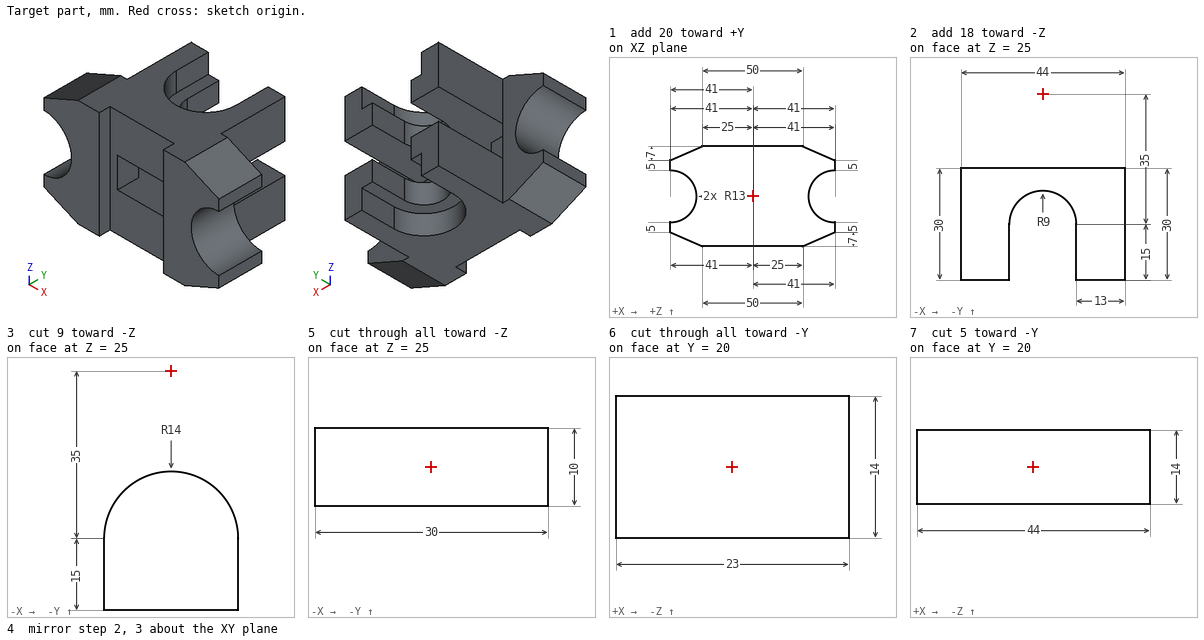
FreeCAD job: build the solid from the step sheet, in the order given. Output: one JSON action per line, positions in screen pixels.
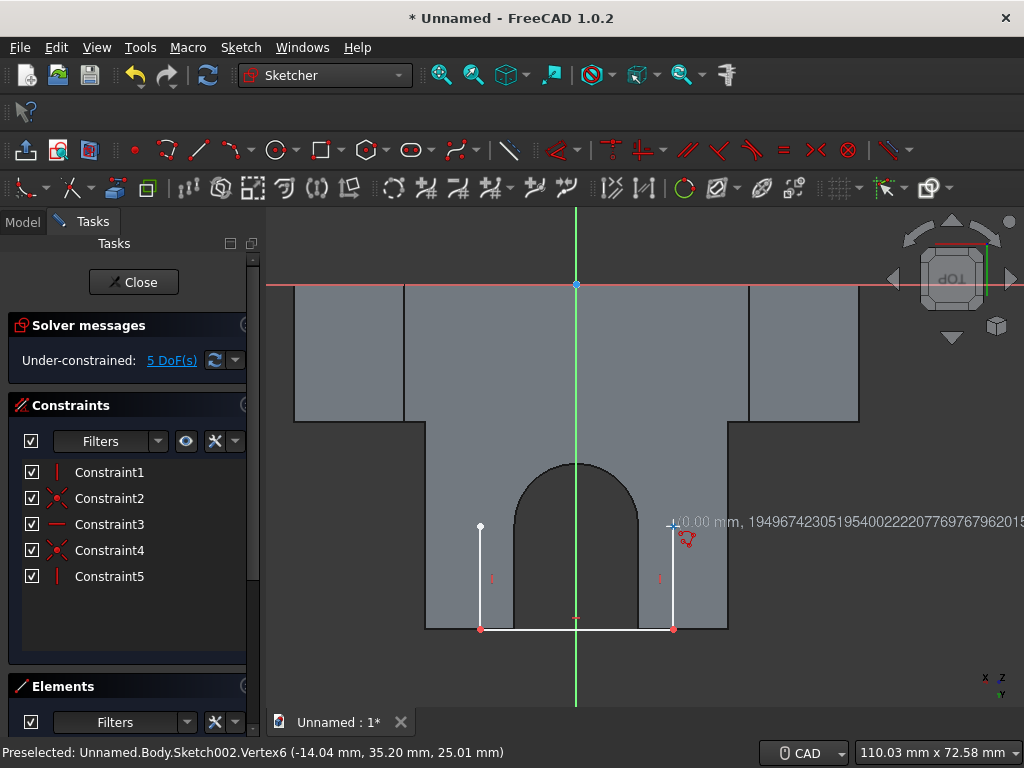
{"action": "left_click", "coordinate": [232, 150]}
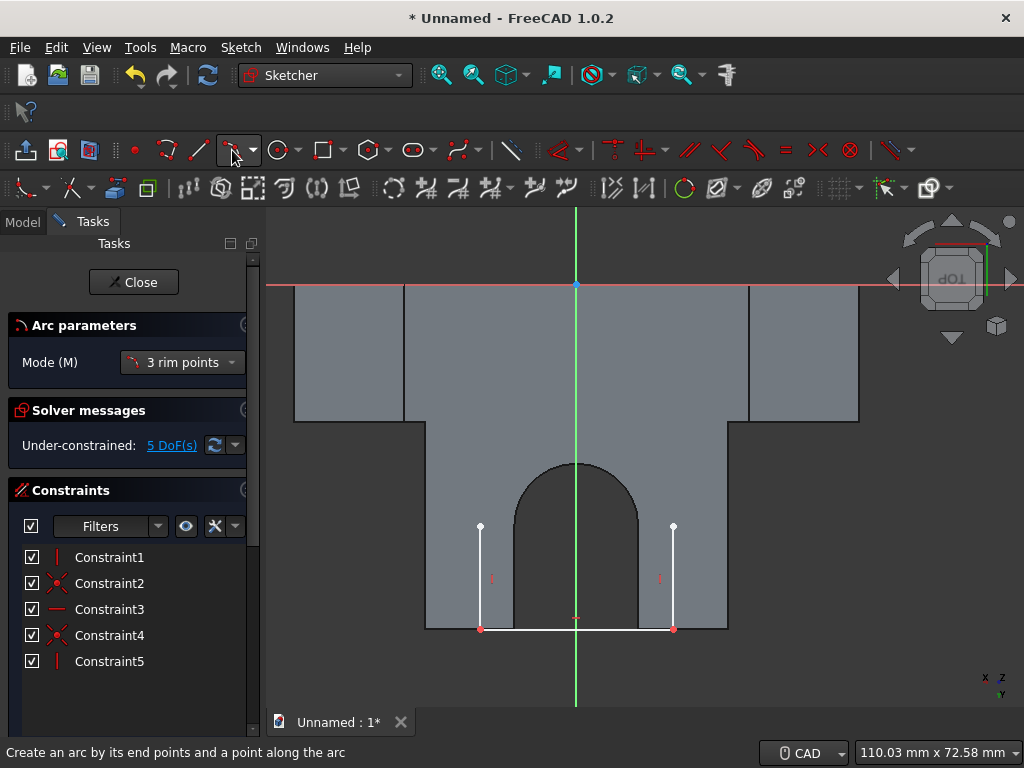
{"action": "left_click", "coordinate": [673, 527]}
{"action": "left_click", "coordinate": [480, 527]}
{"action": "left_click", "coordinate": [606, 434]}
{"action": "key", "text": "Escape"}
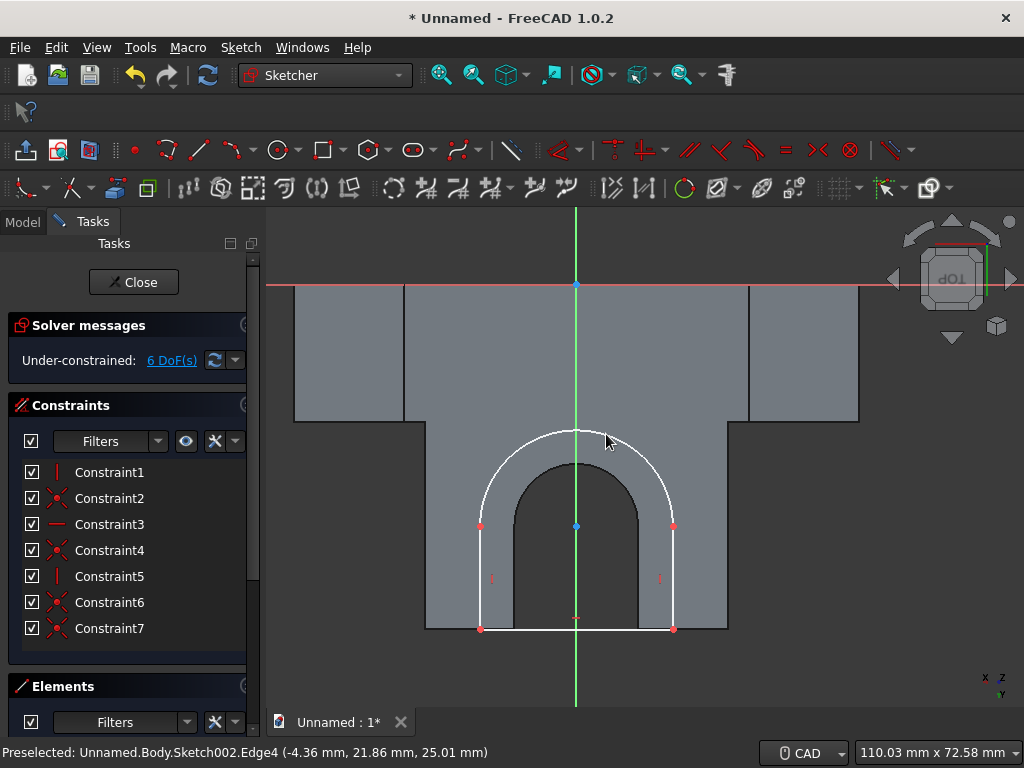
{"action": "left_click", "coordinate": [480, 558]}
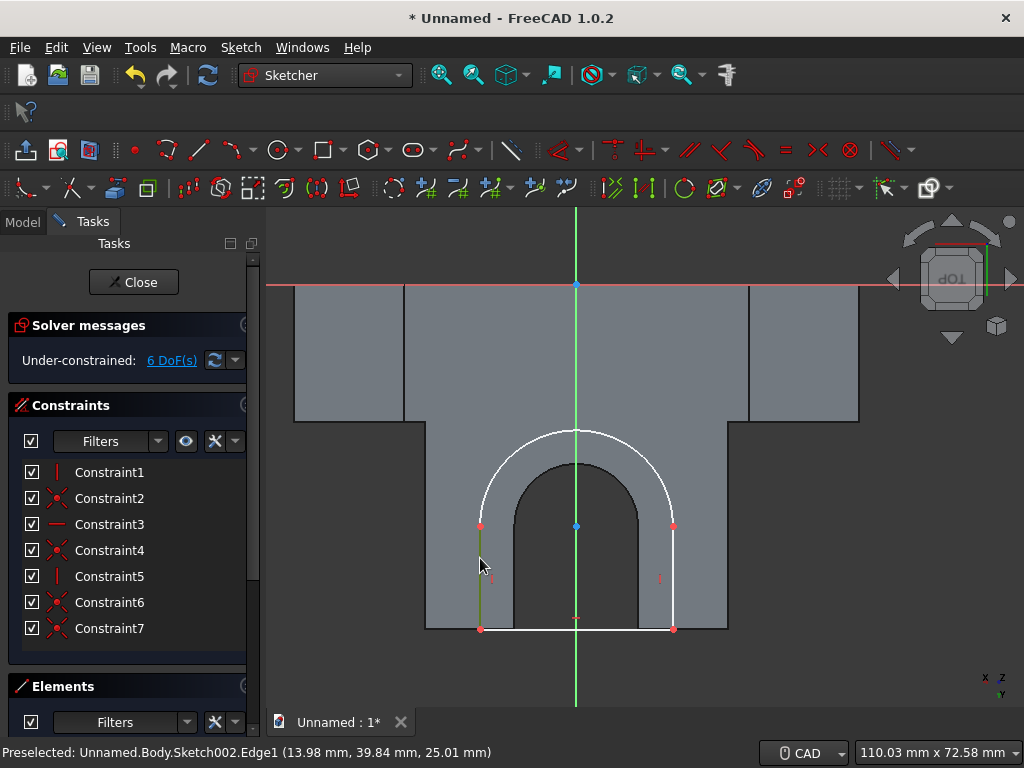
{"action": "left_click", "coordinate": [633, 449]}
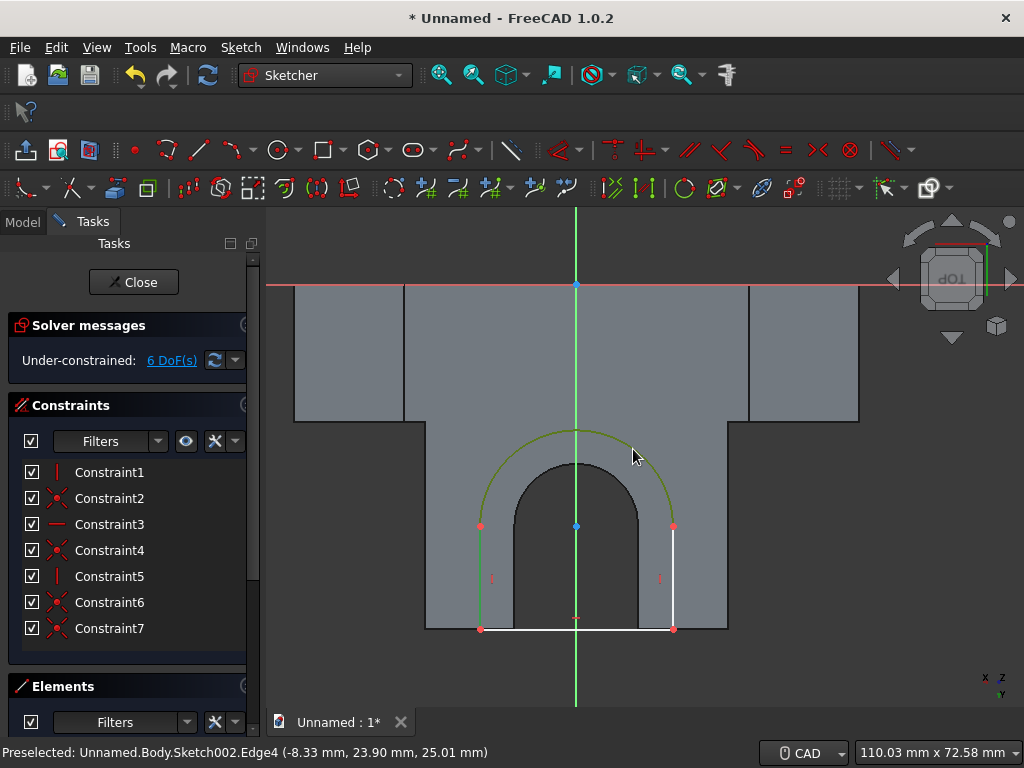
{"action": "left_click", "coordinate": [754, 150]}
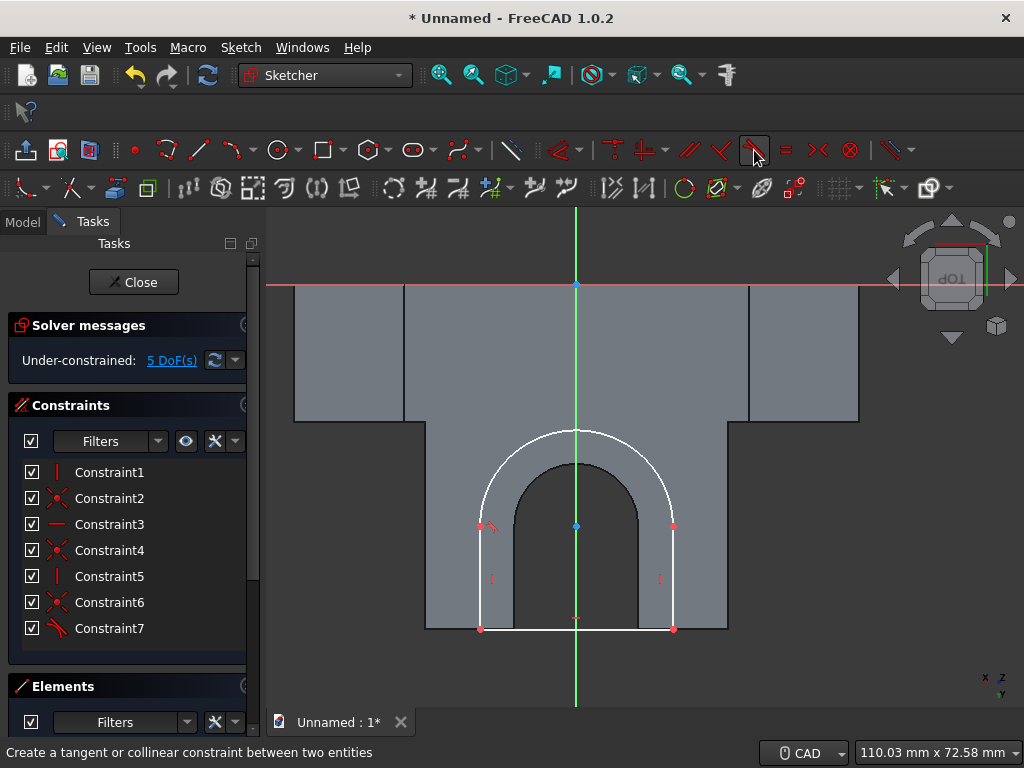
{"action": "left_click", "coordinate": [673, 599]}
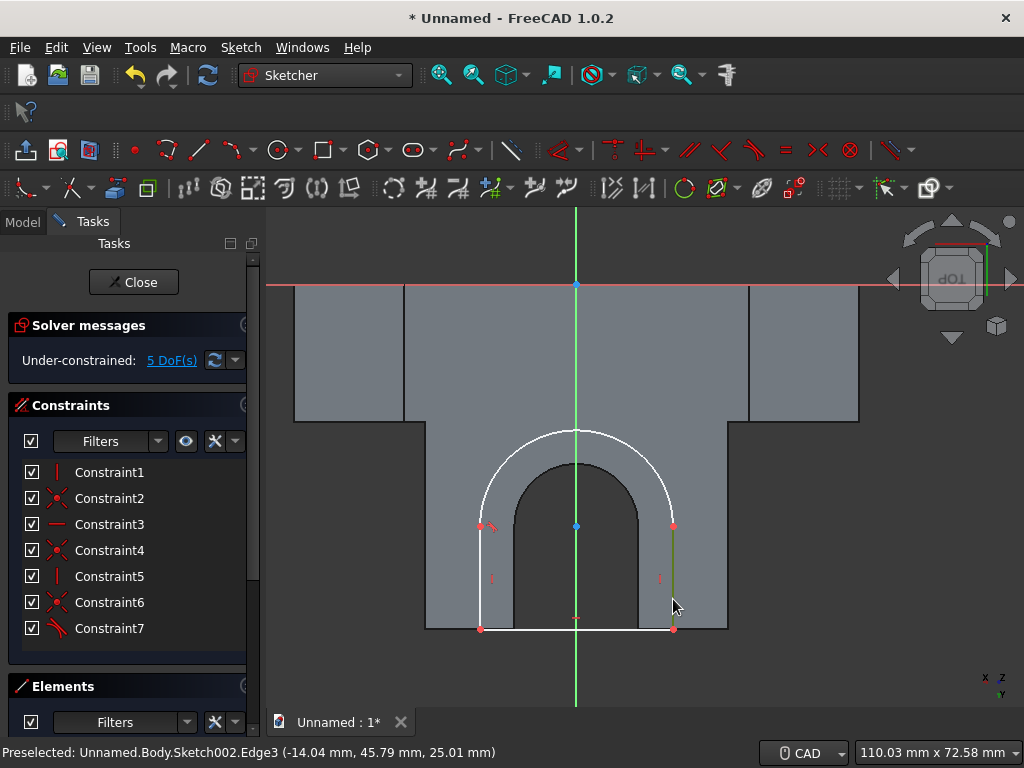
{"action": "left_click", "coordinate": [633, 449]}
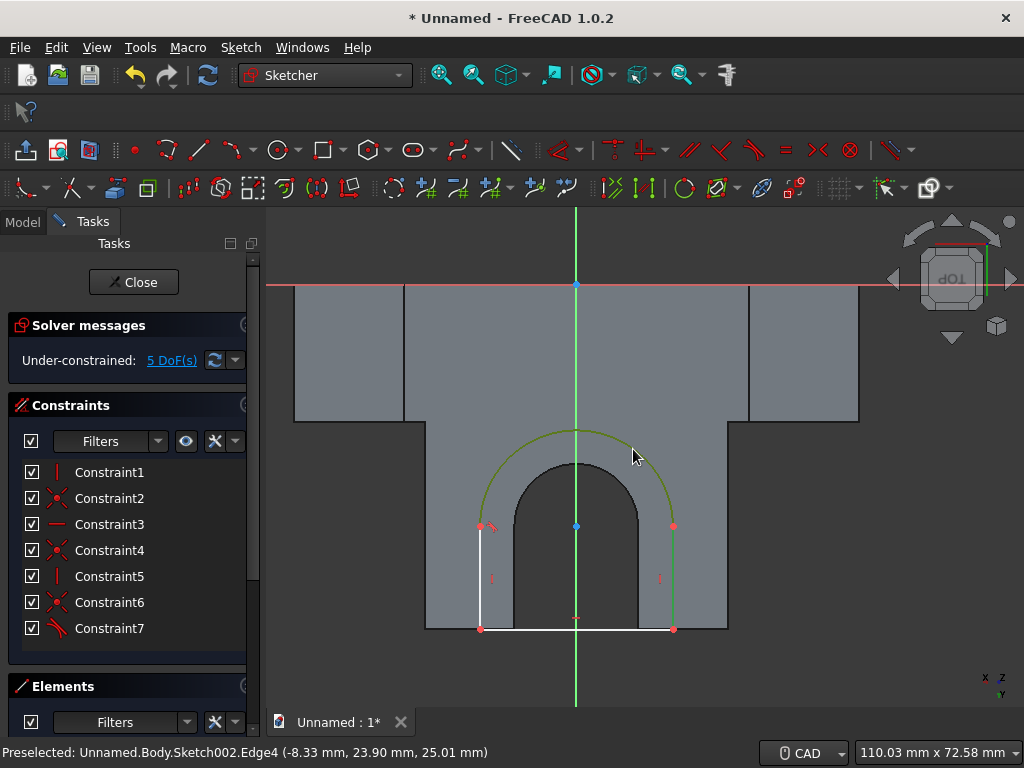
{"action": "left_click", "coordinate": [754, 150]}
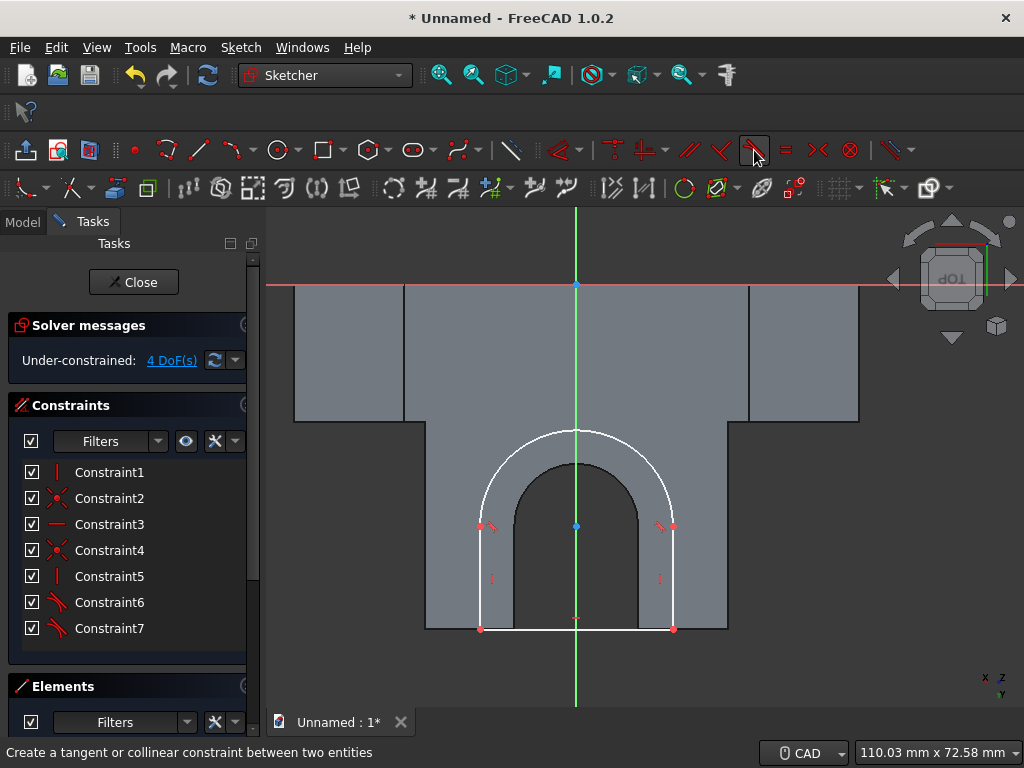
{"action": "left_click", "coordinate": [577, 527]}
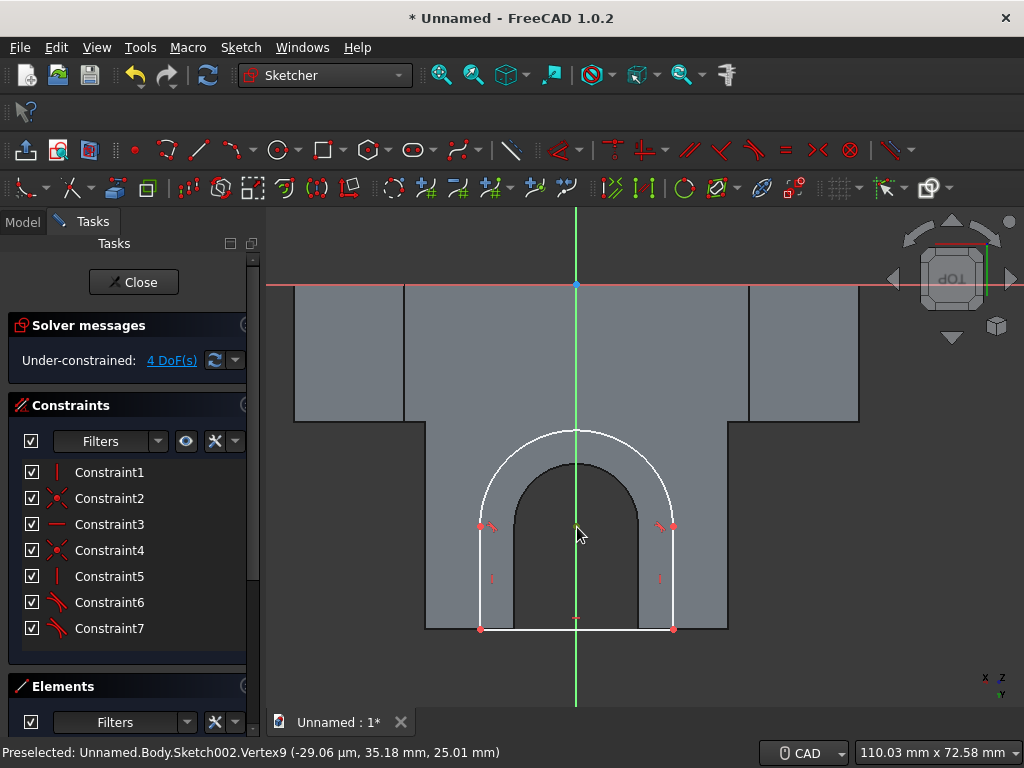
{"action": "left_click", "coordinate": [576, 584]}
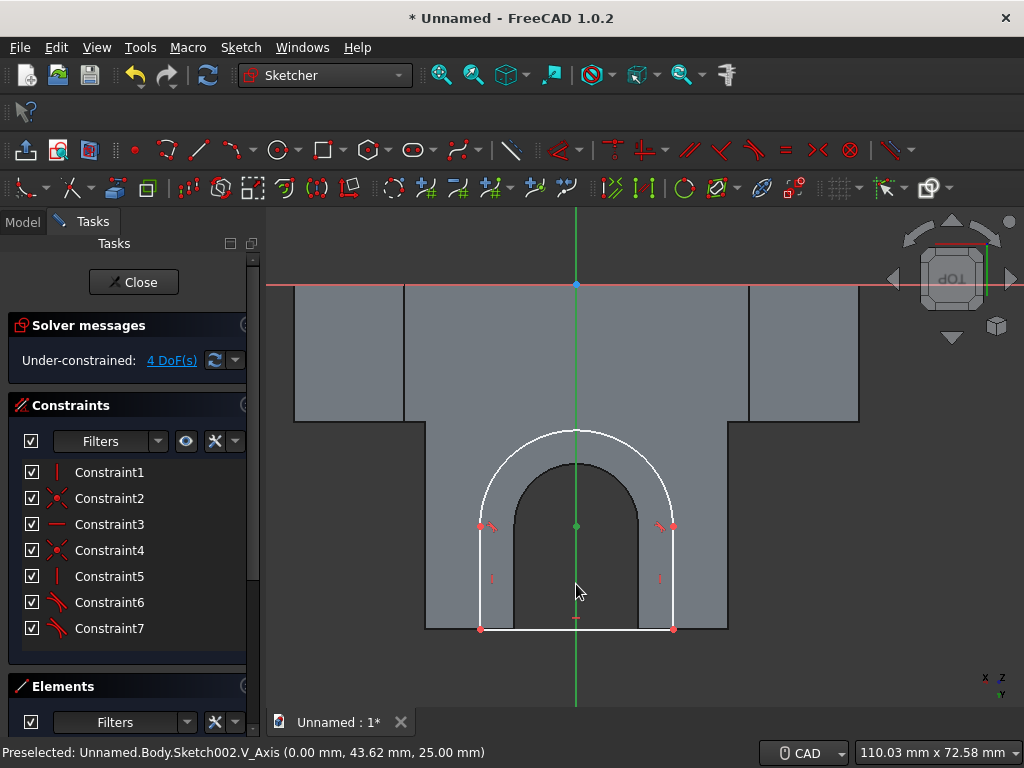
{"action": "left_click", "coordinate": [614, 150]}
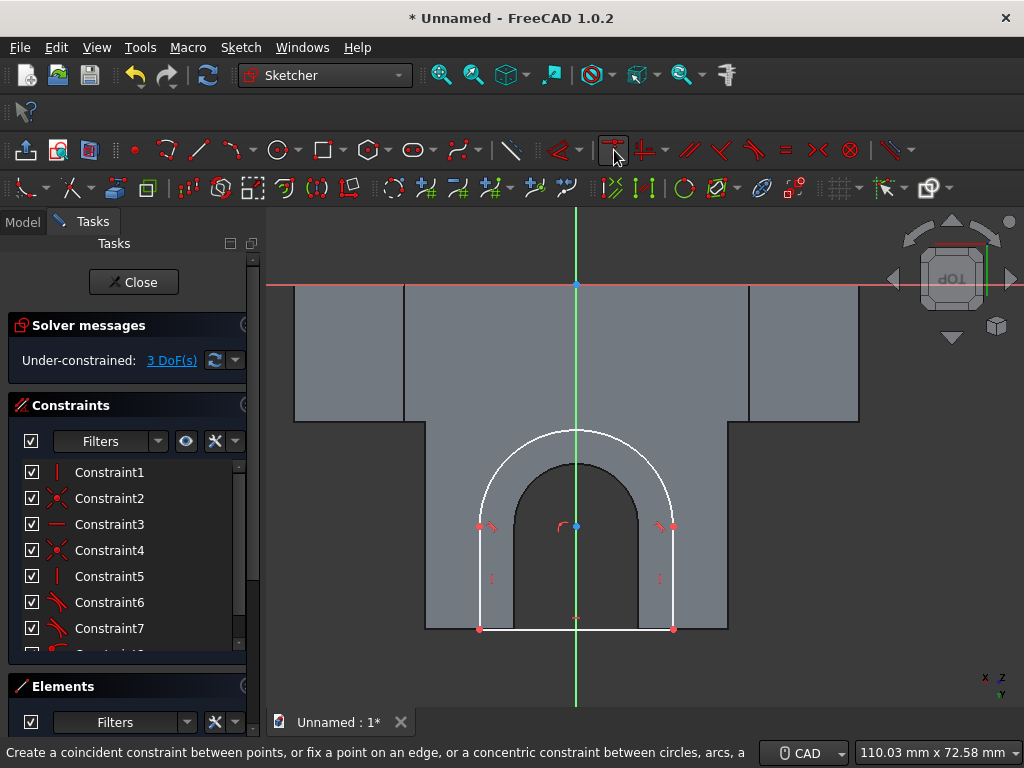
{"action": "left_click", "coordinate": [558, 150]}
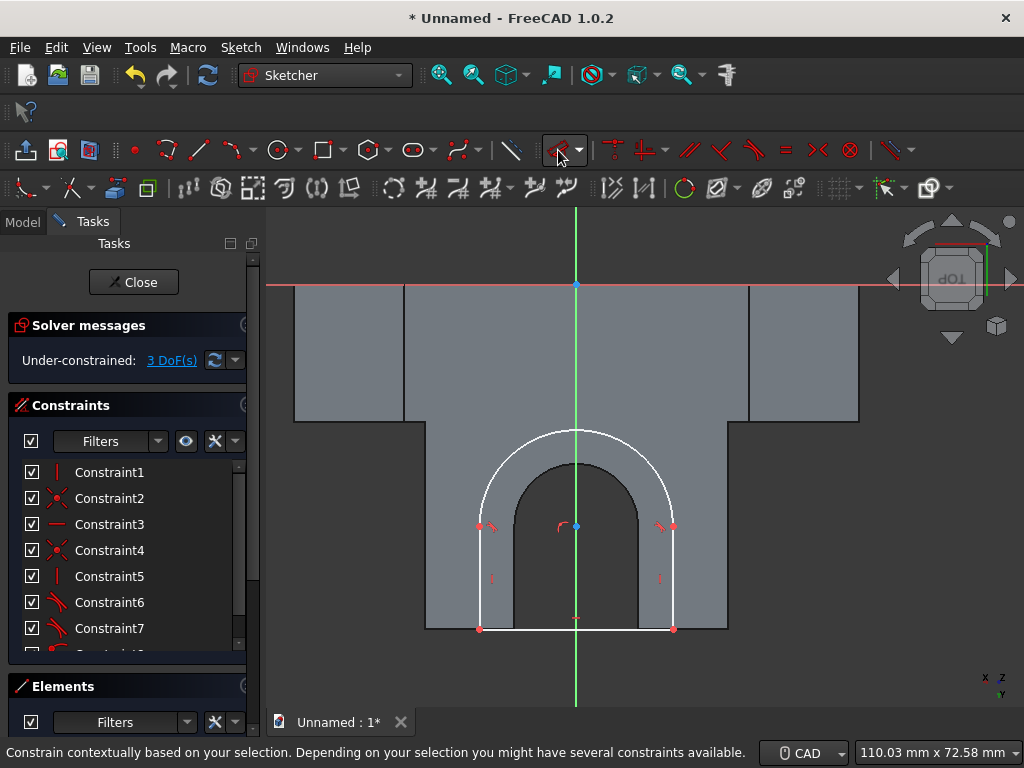
{"action": "left_click", "coordinate": [633, 449]}
{"action": "left_click", "coordinate": [652, 423]}